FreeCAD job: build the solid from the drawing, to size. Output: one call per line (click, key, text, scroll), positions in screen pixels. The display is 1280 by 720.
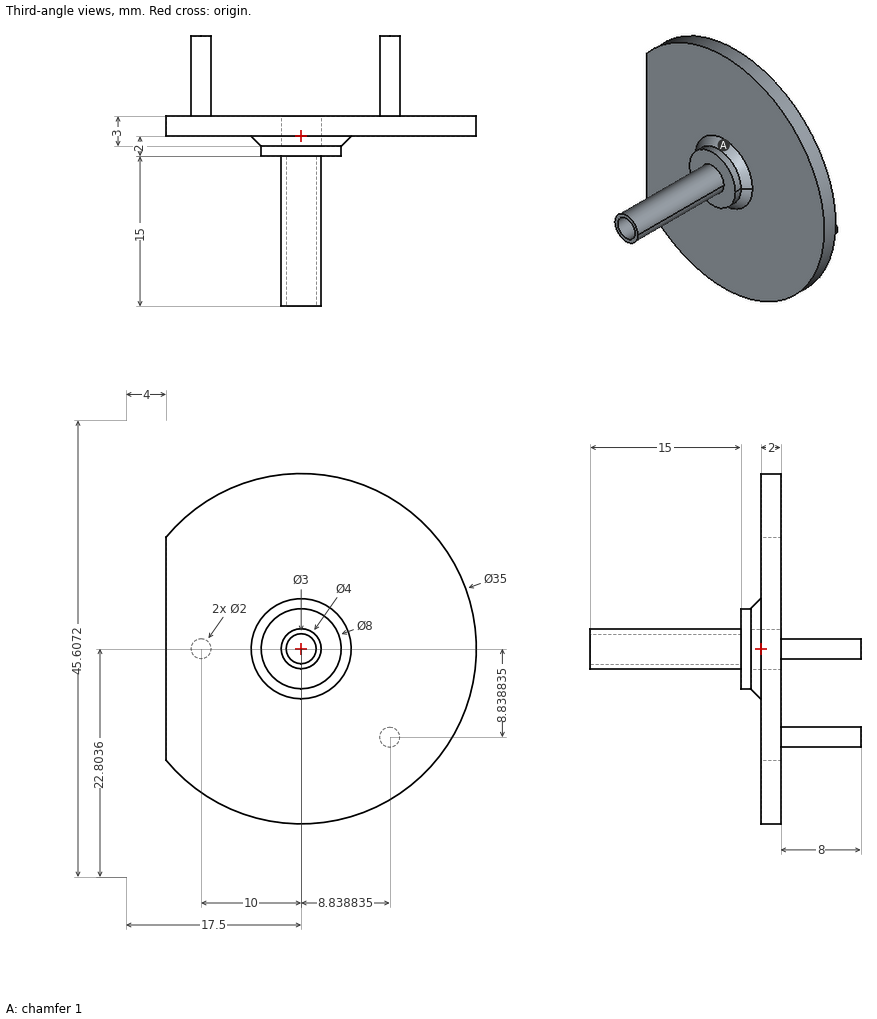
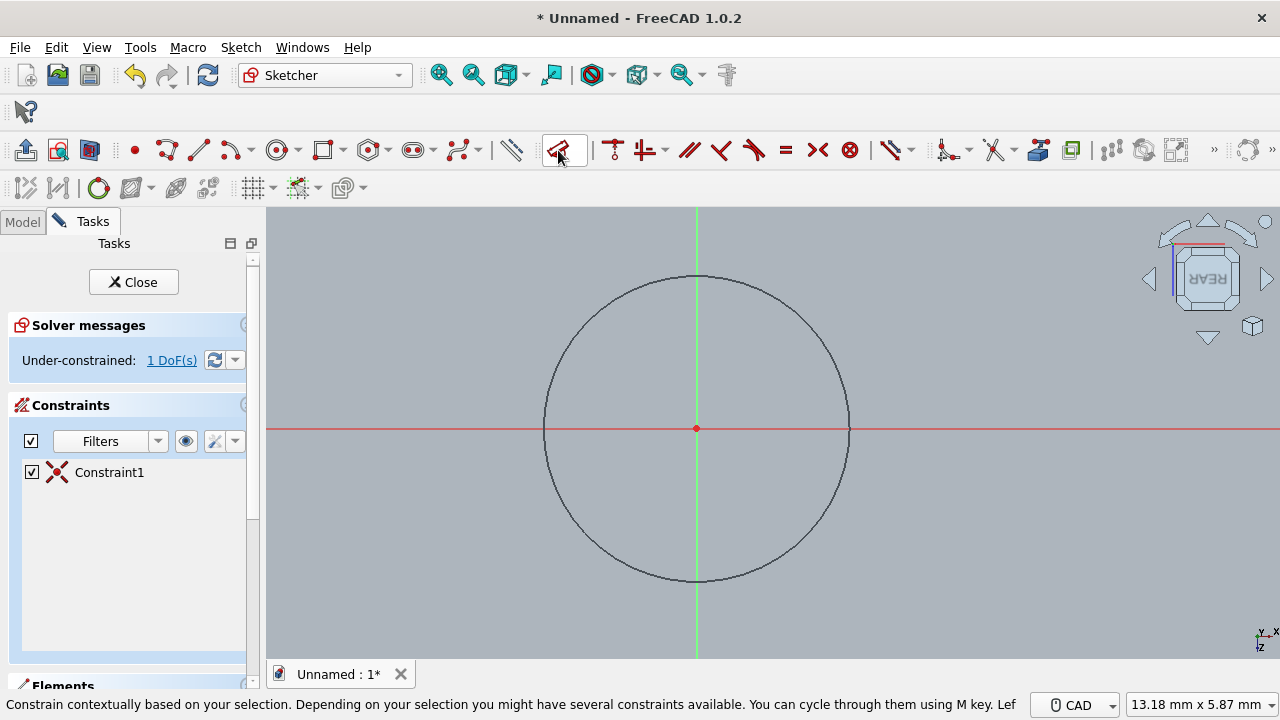
click(804, 320)
click(826, 297)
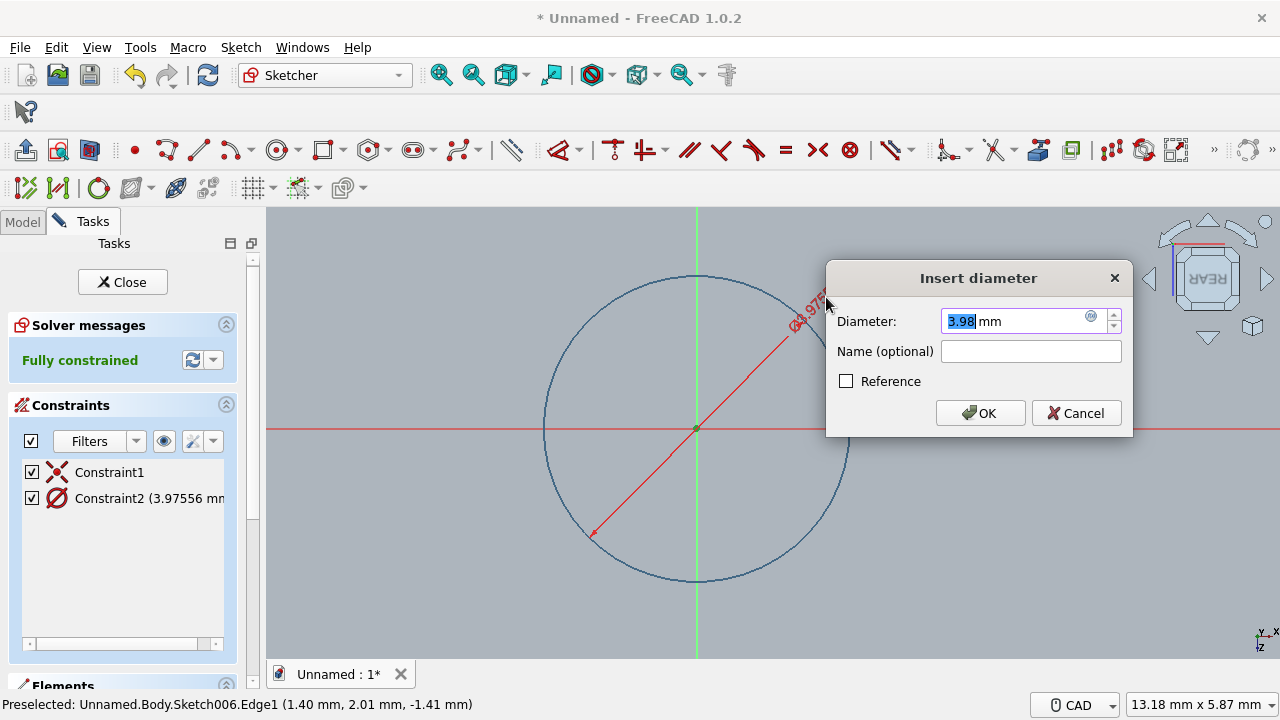
text(4)
key(Return)
key(Escape)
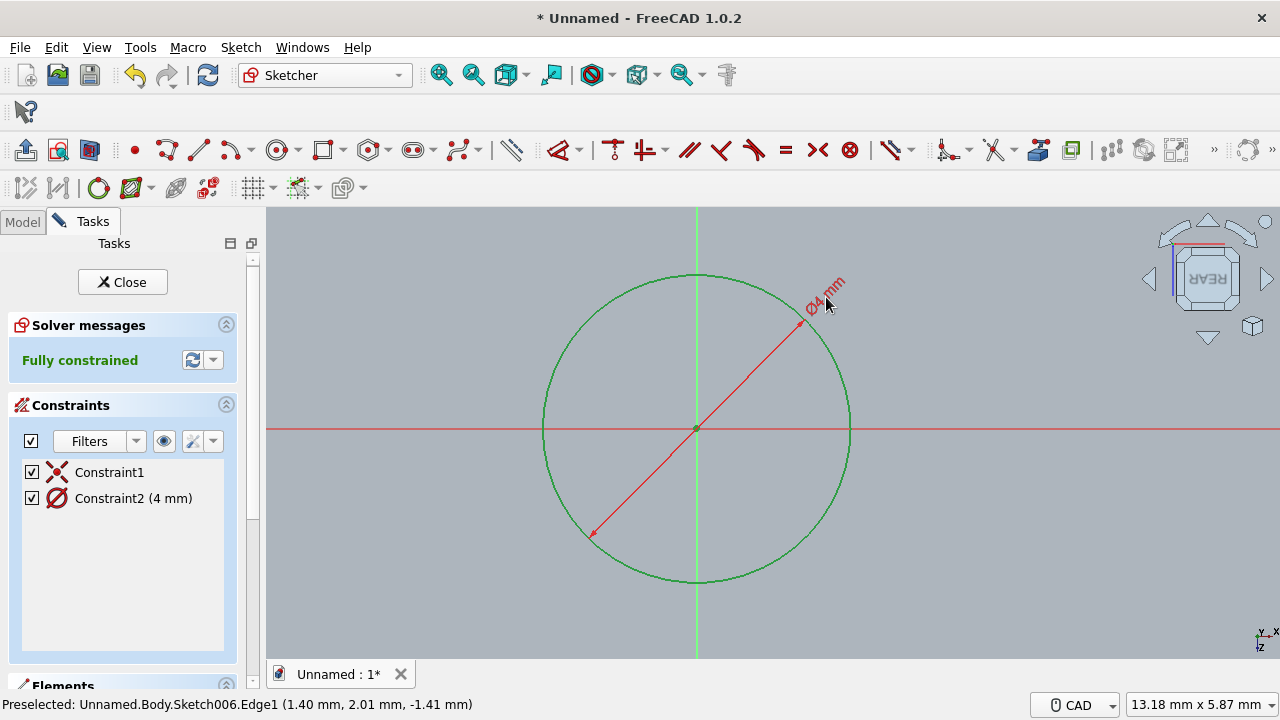
click(123, 282)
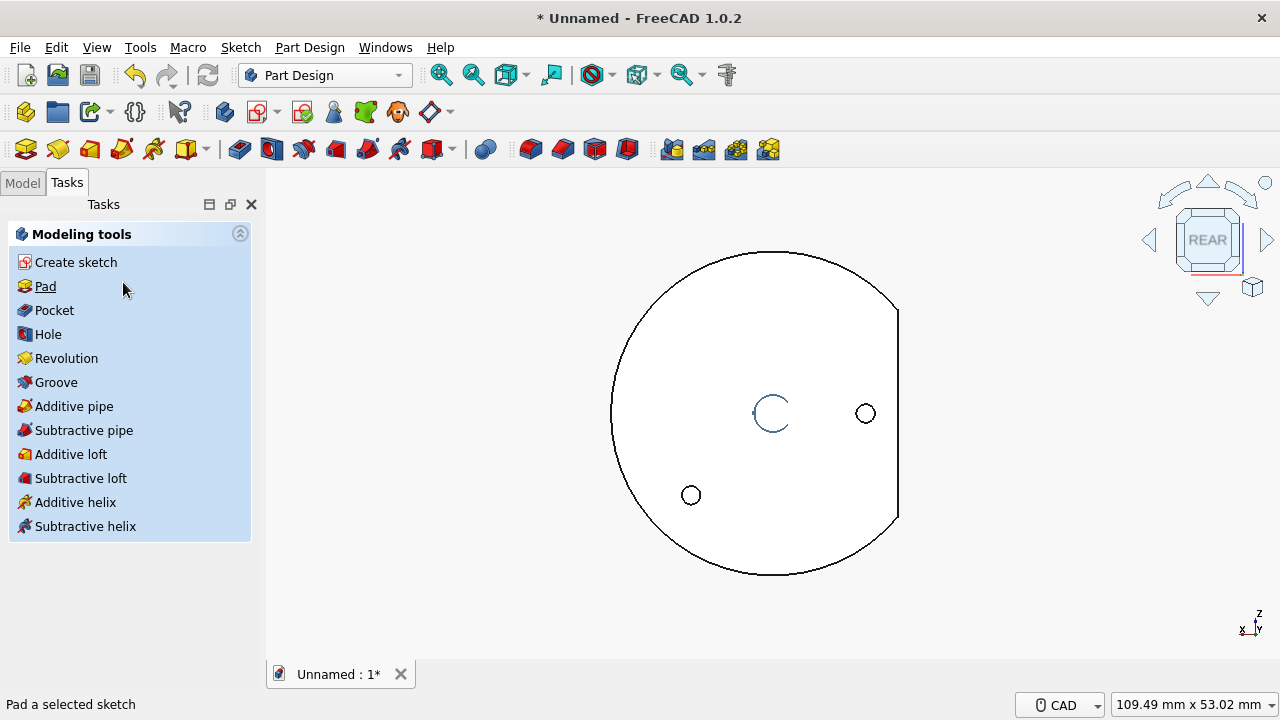
click(240, 150)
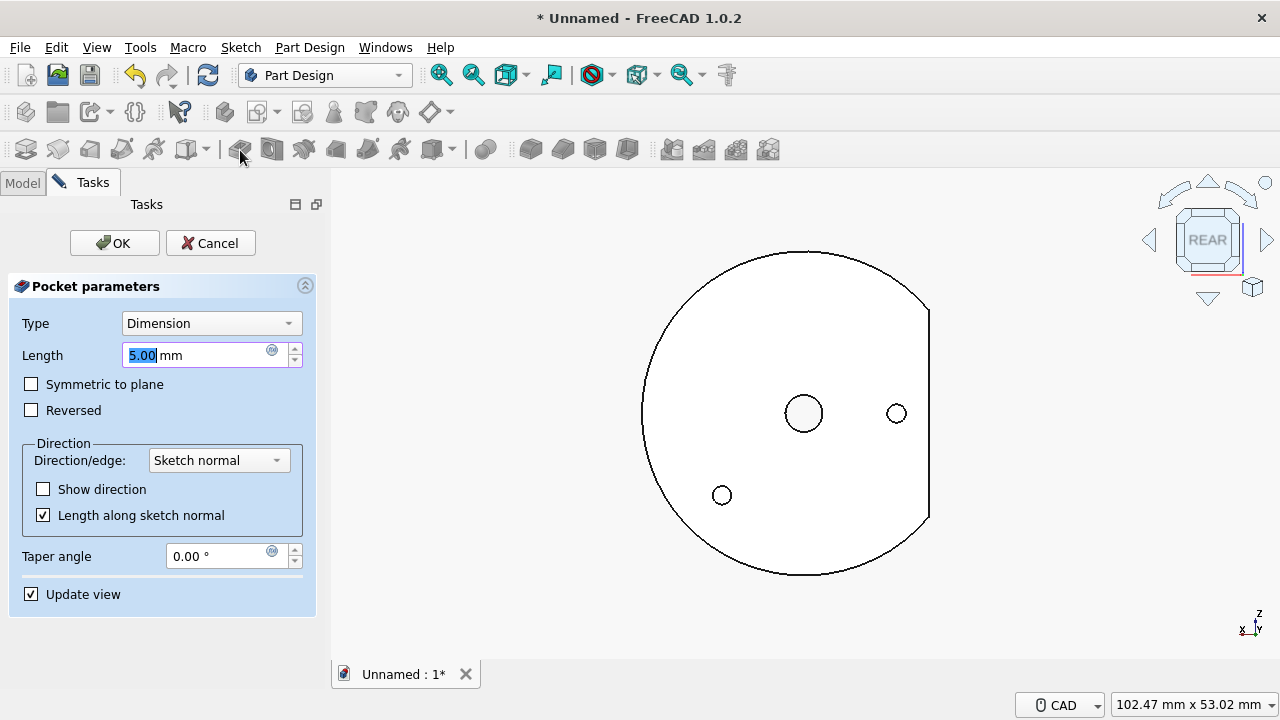
text(3)
key(Tab)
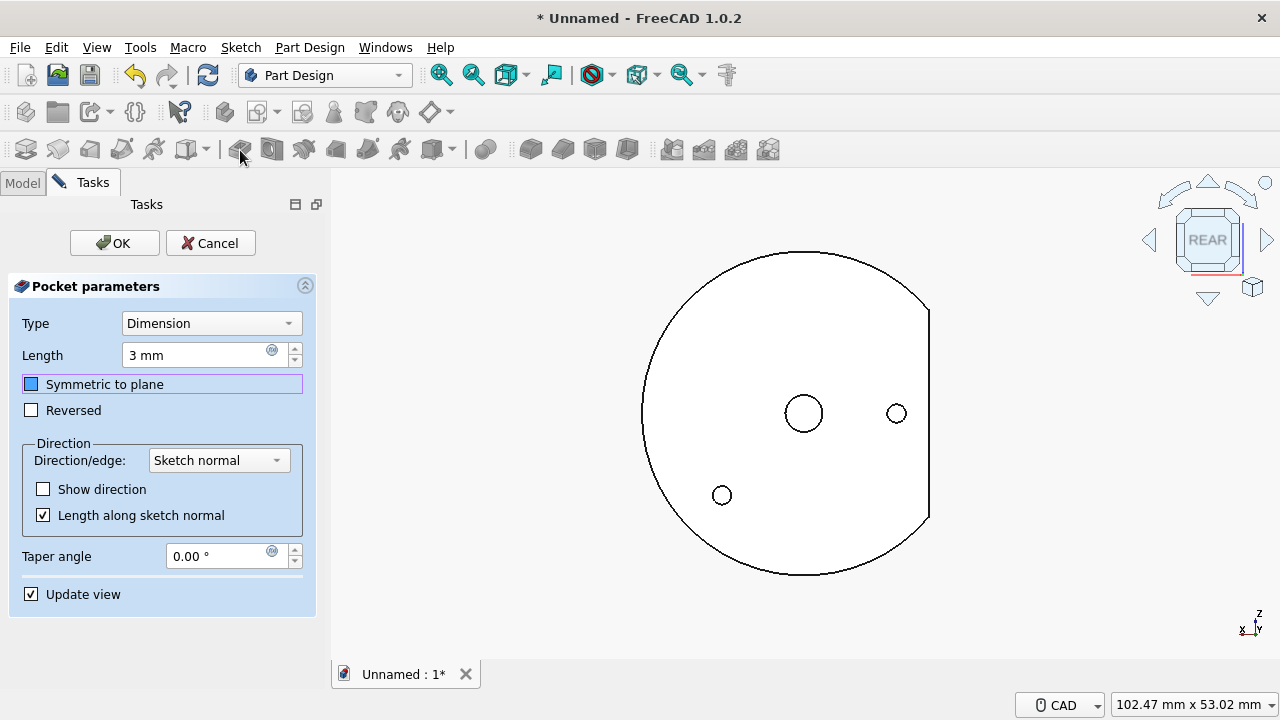
click(115, 243)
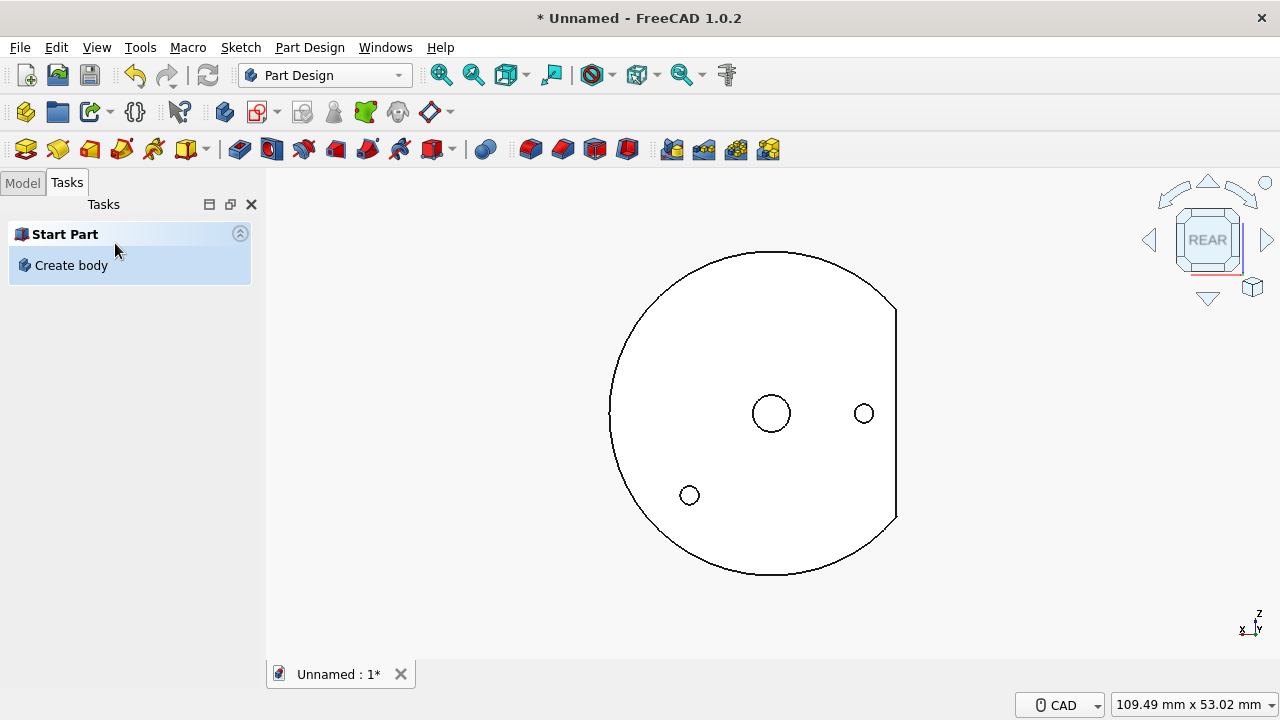
key(0)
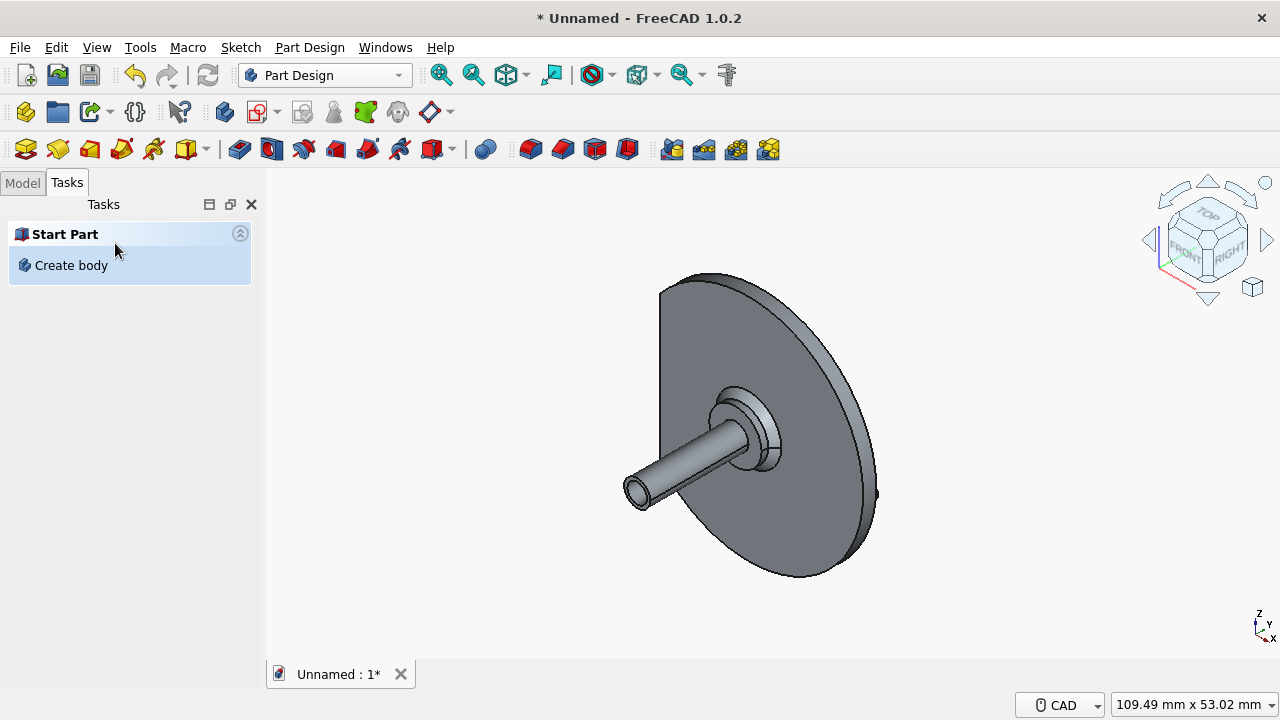
click(442, 76)